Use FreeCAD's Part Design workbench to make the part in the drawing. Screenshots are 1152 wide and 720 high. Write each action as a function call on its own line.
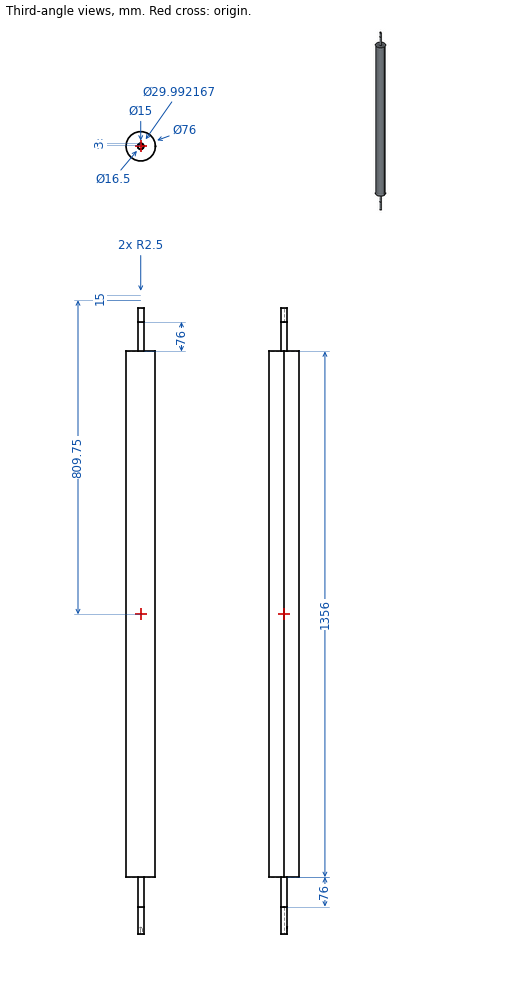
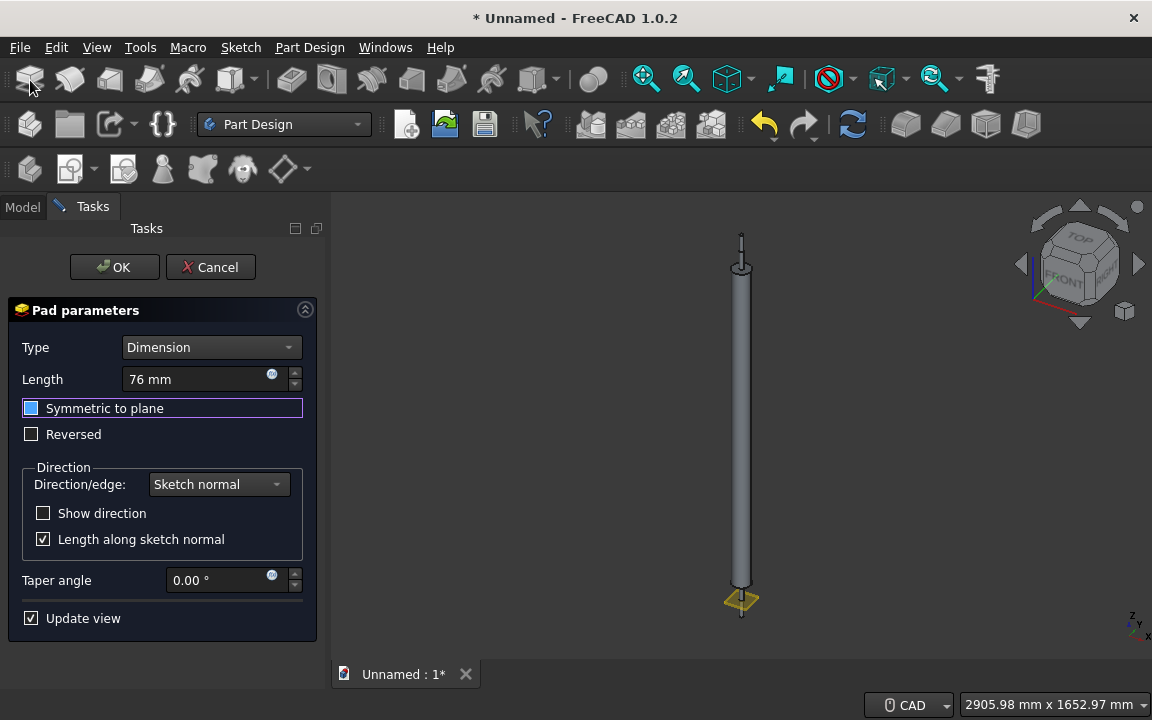
click(115, 267)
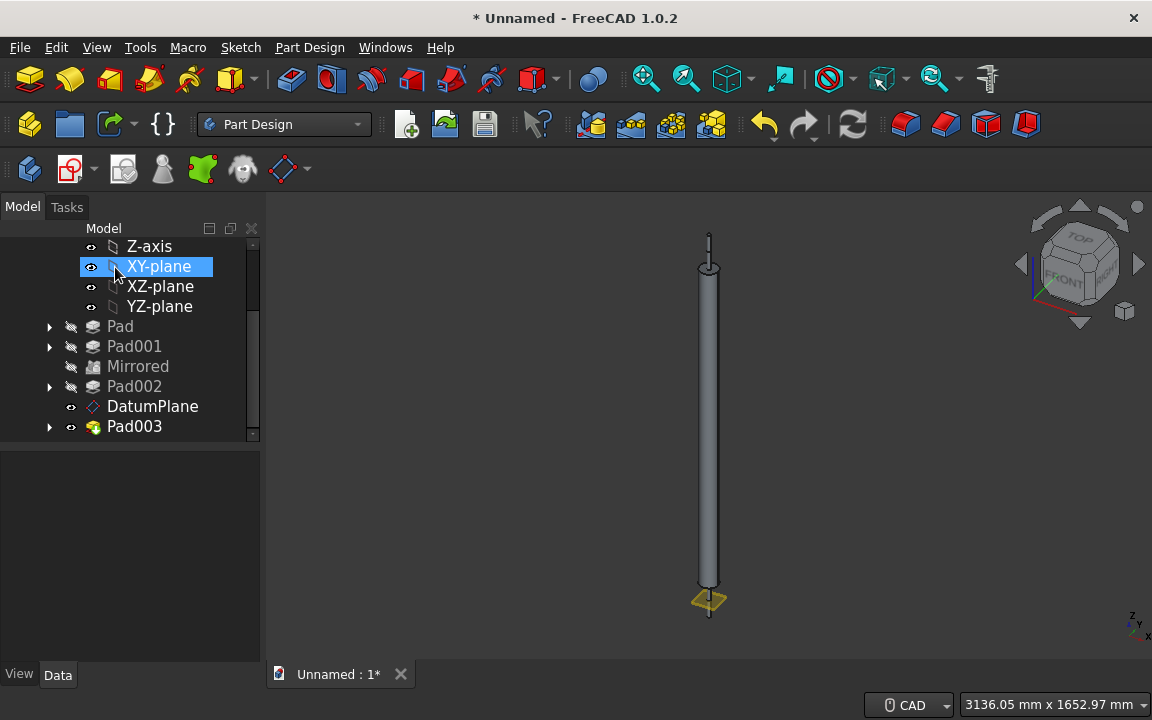
click(116, 407)
key(space)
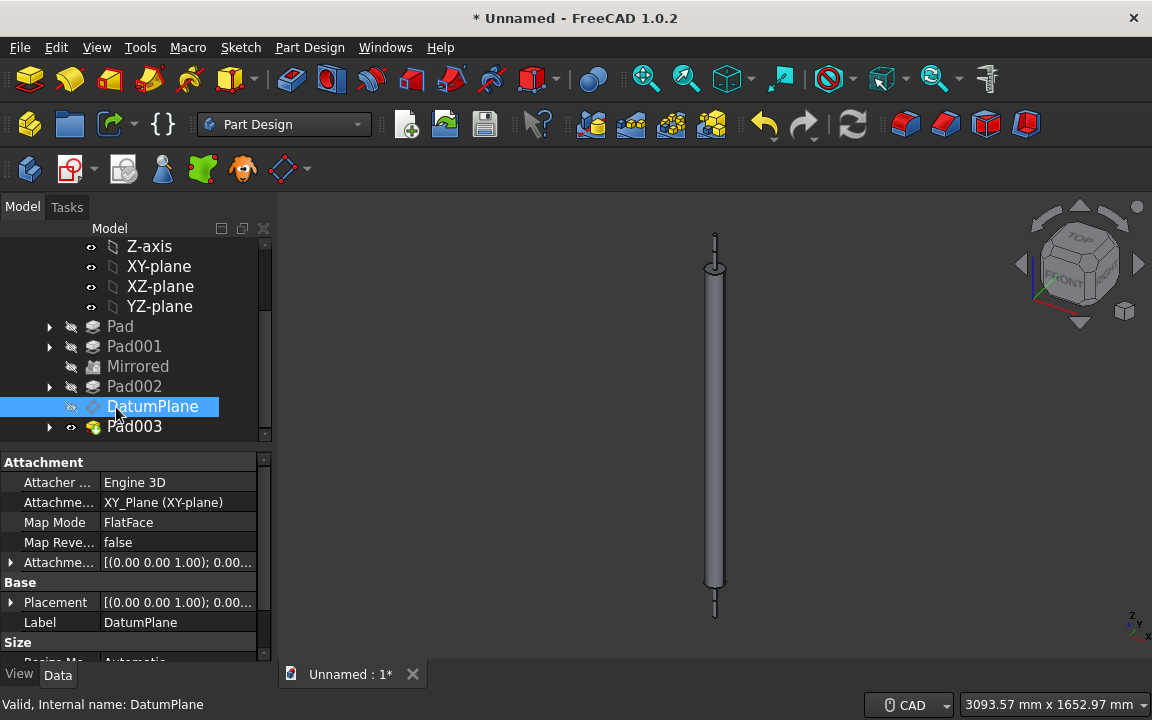
scroll(160, 342, down, 3)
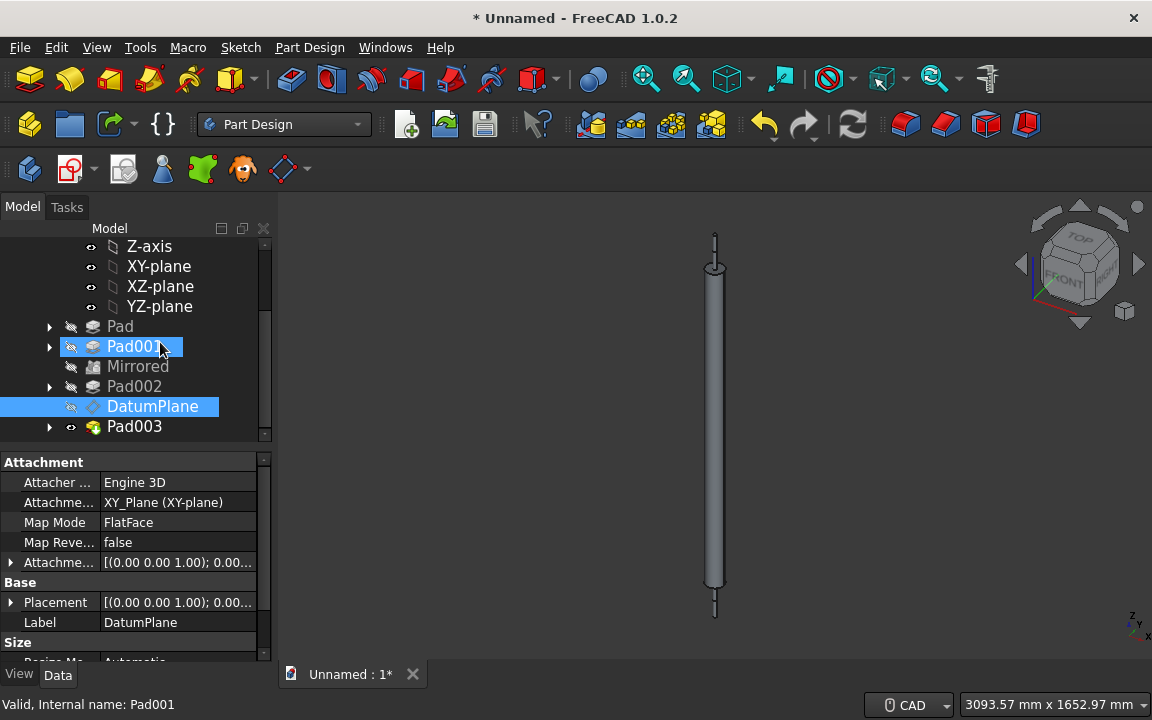
scroll(160, 342, up, 15)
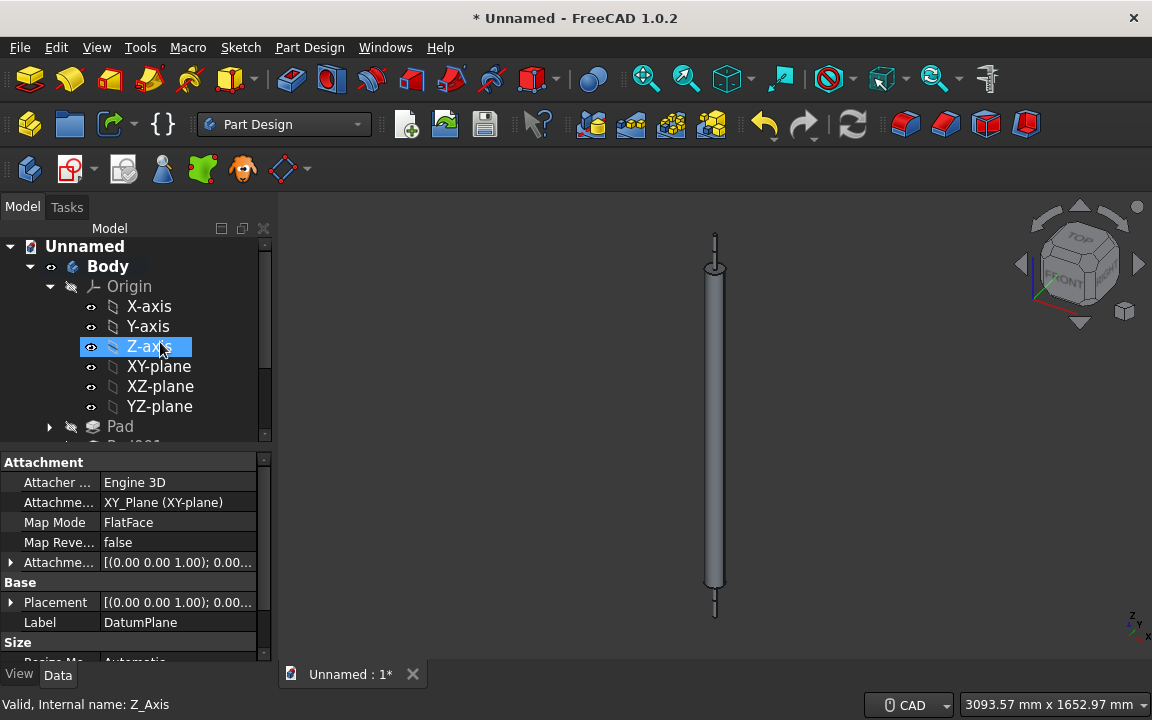
click(136, 387)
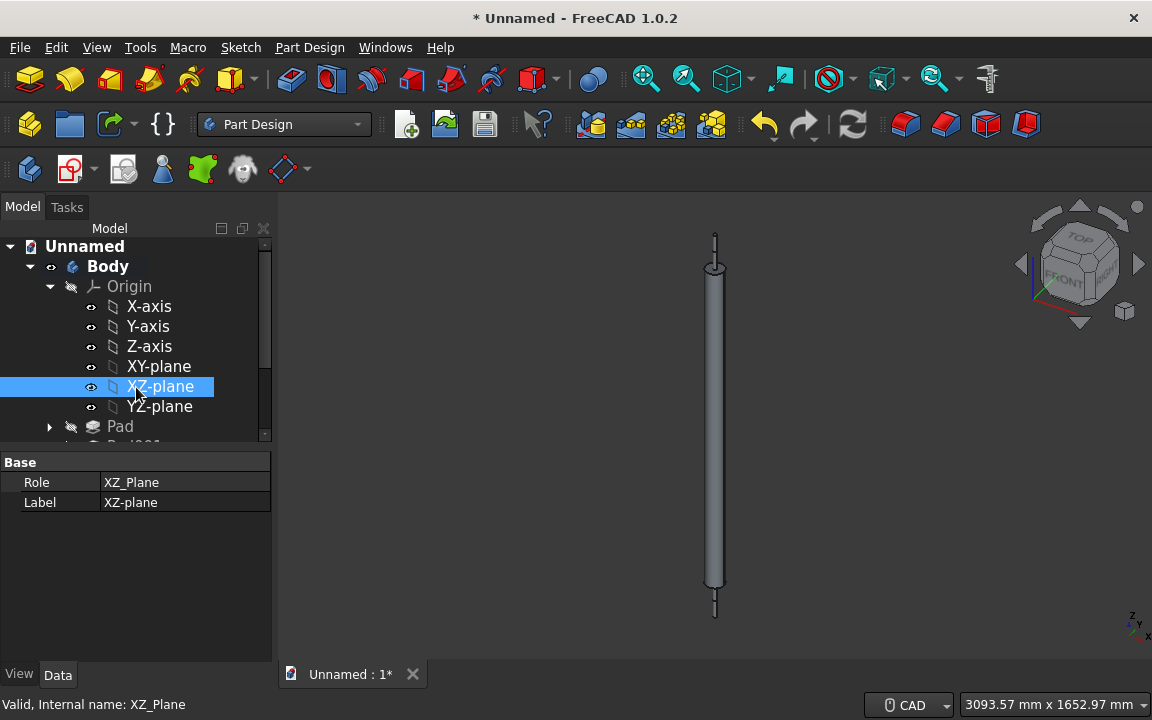
click(284, 170)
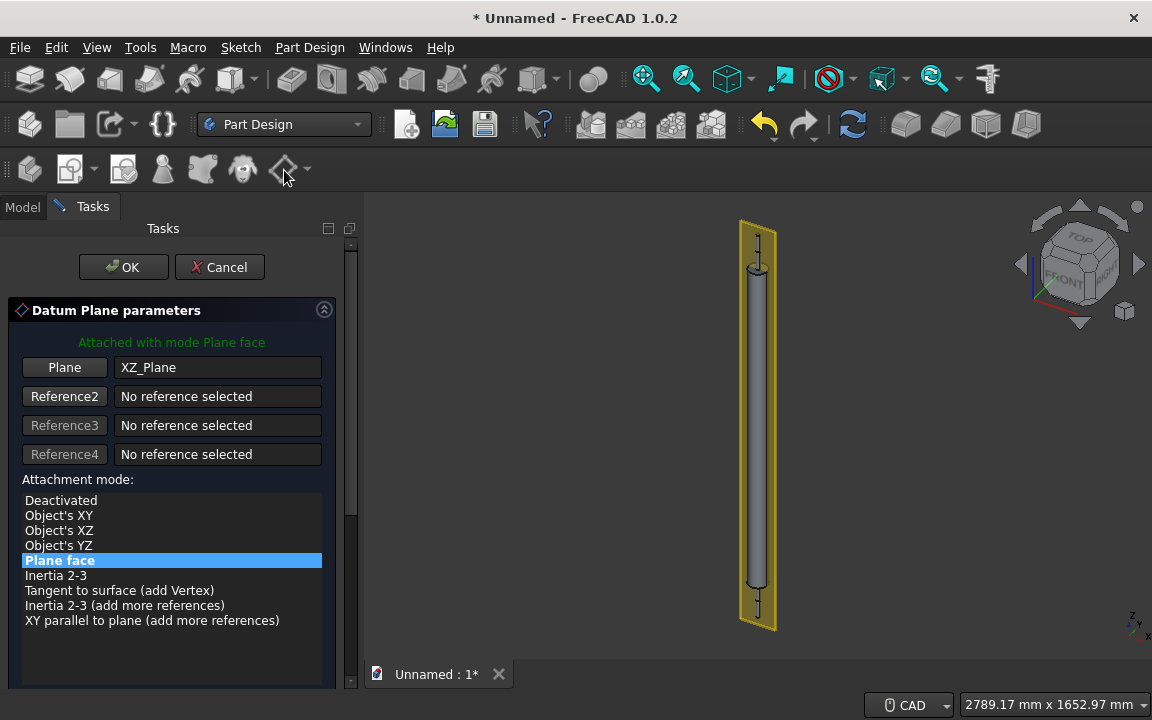
scroll(351, 463, down, 3)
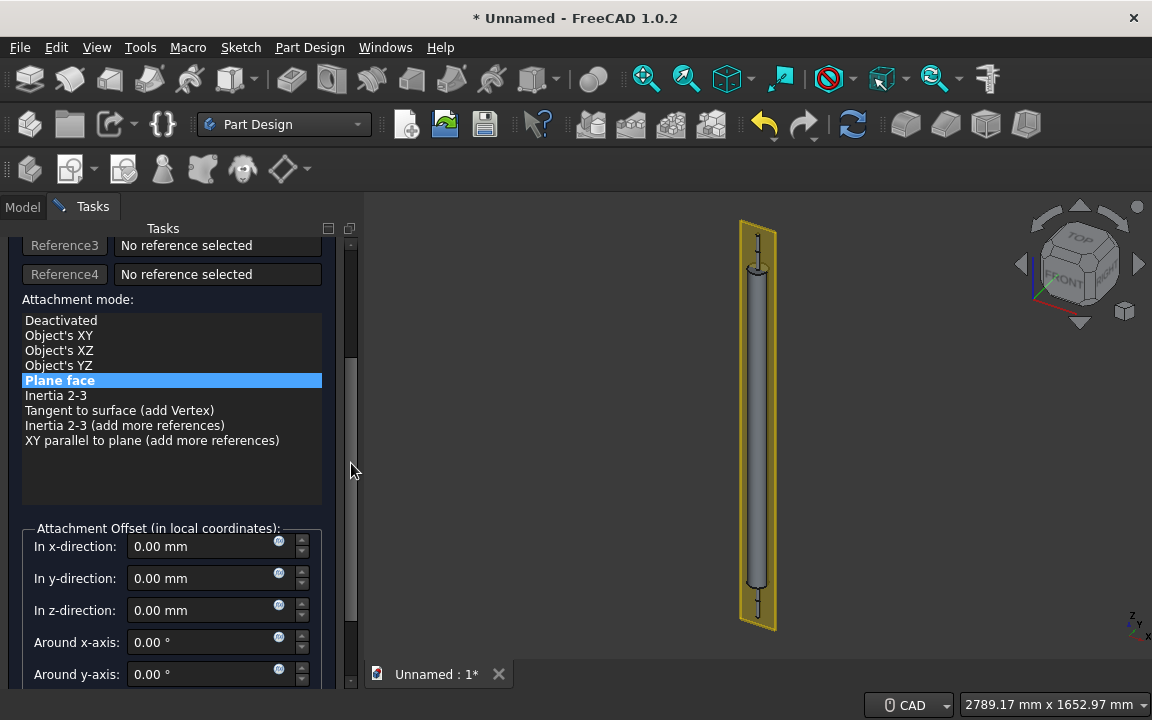
triple_click(210, 610)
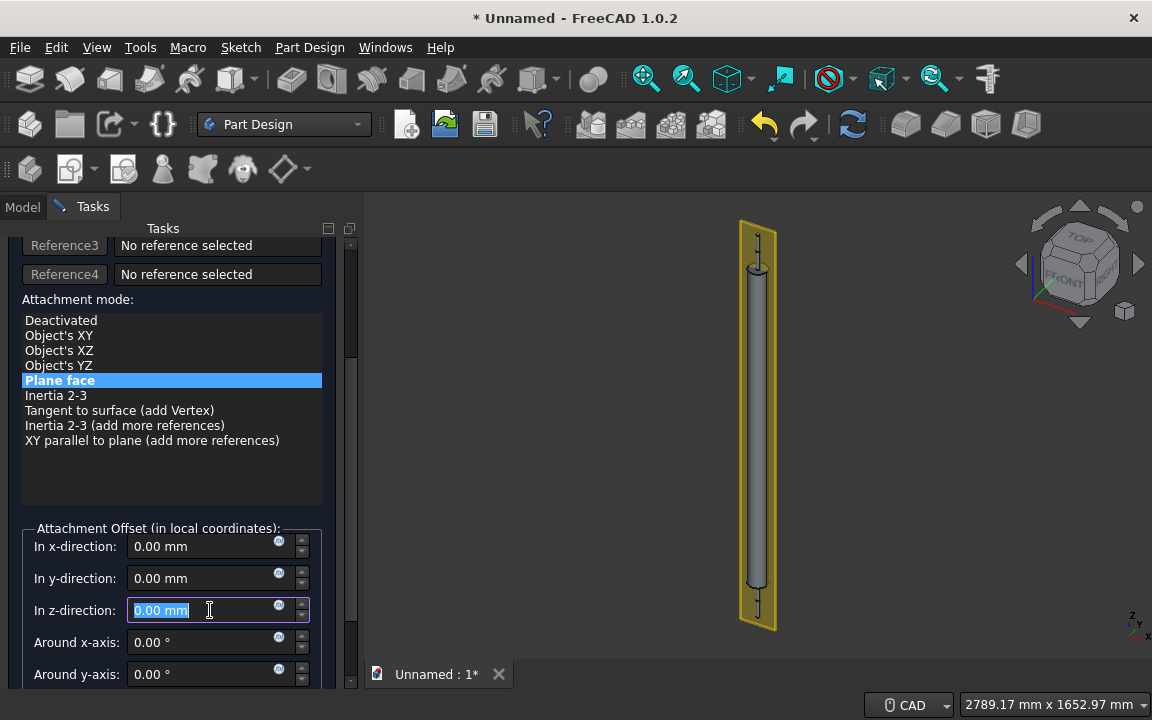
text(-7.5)
key(Tab)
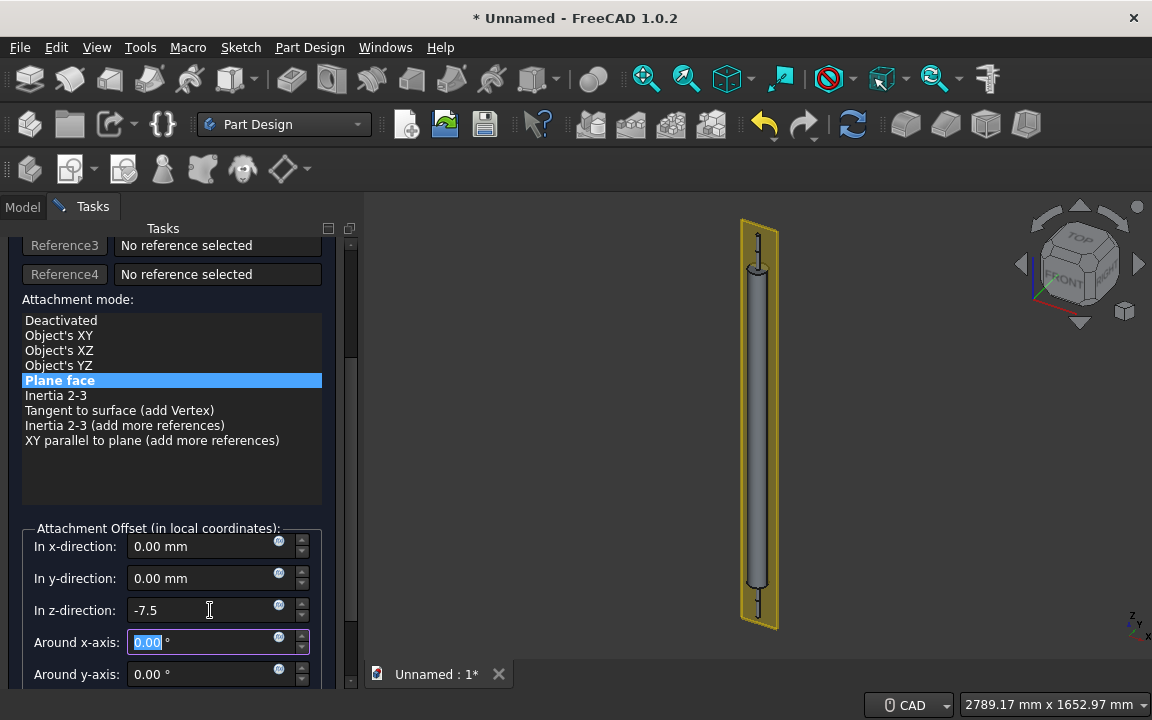
scroll(351, 463, up, 4)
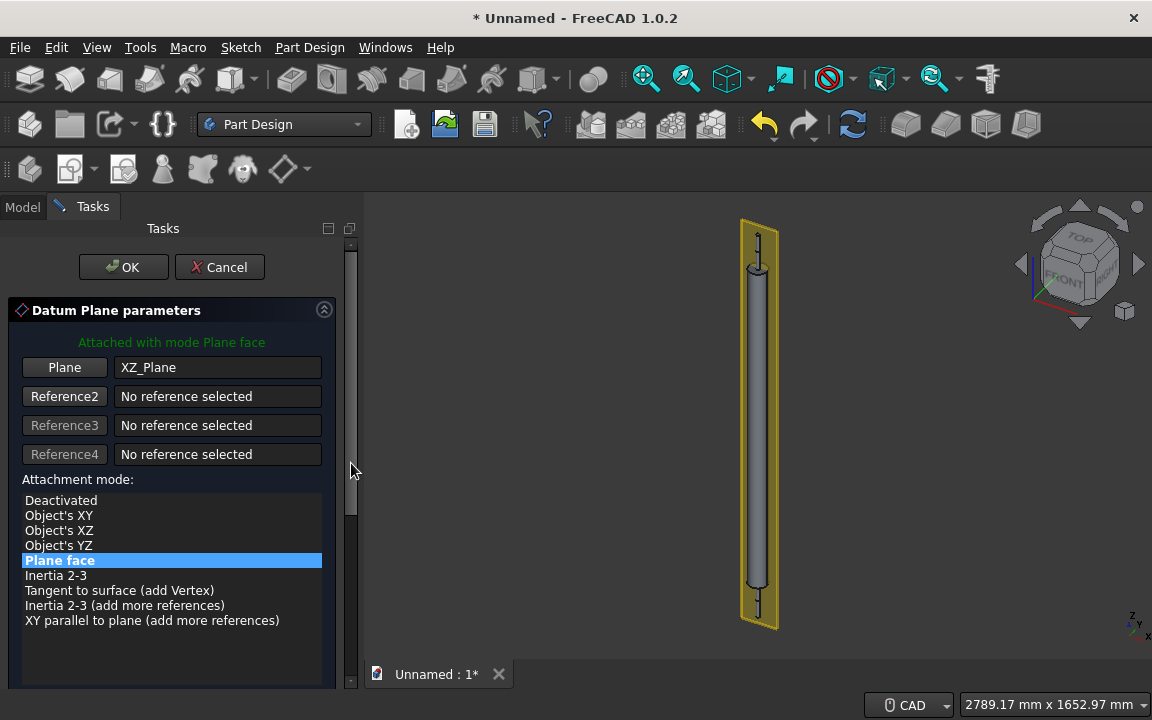
click(124, 267)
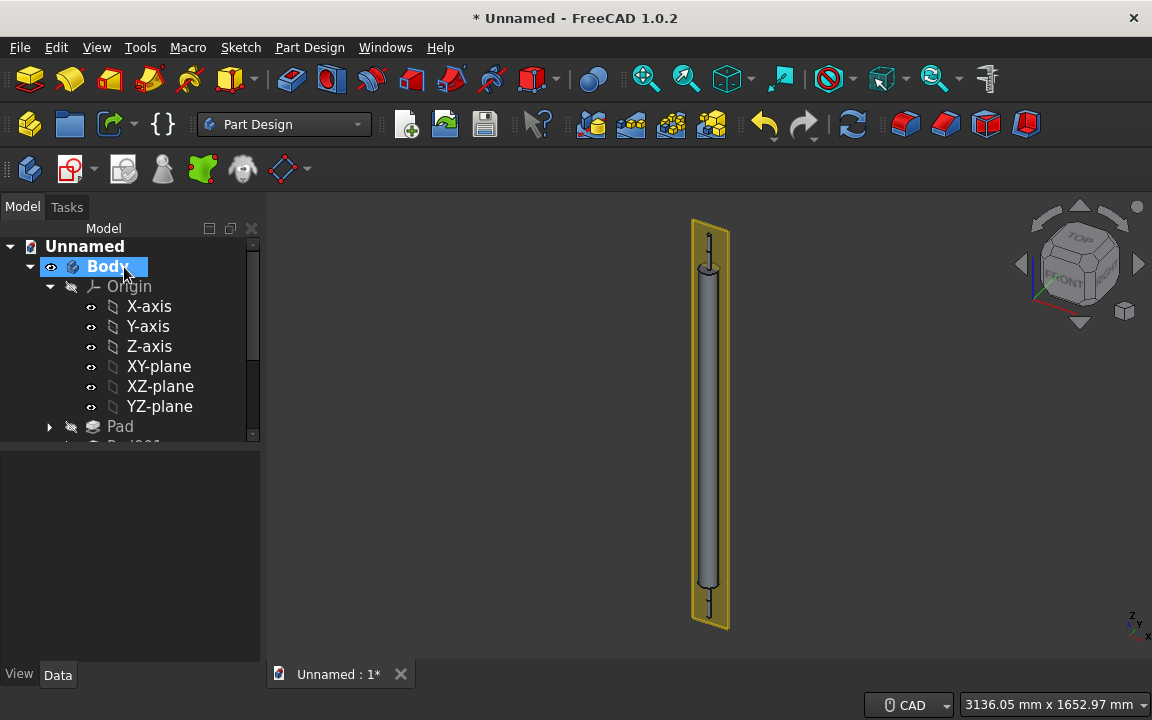
scroll(100, 342, down, 3)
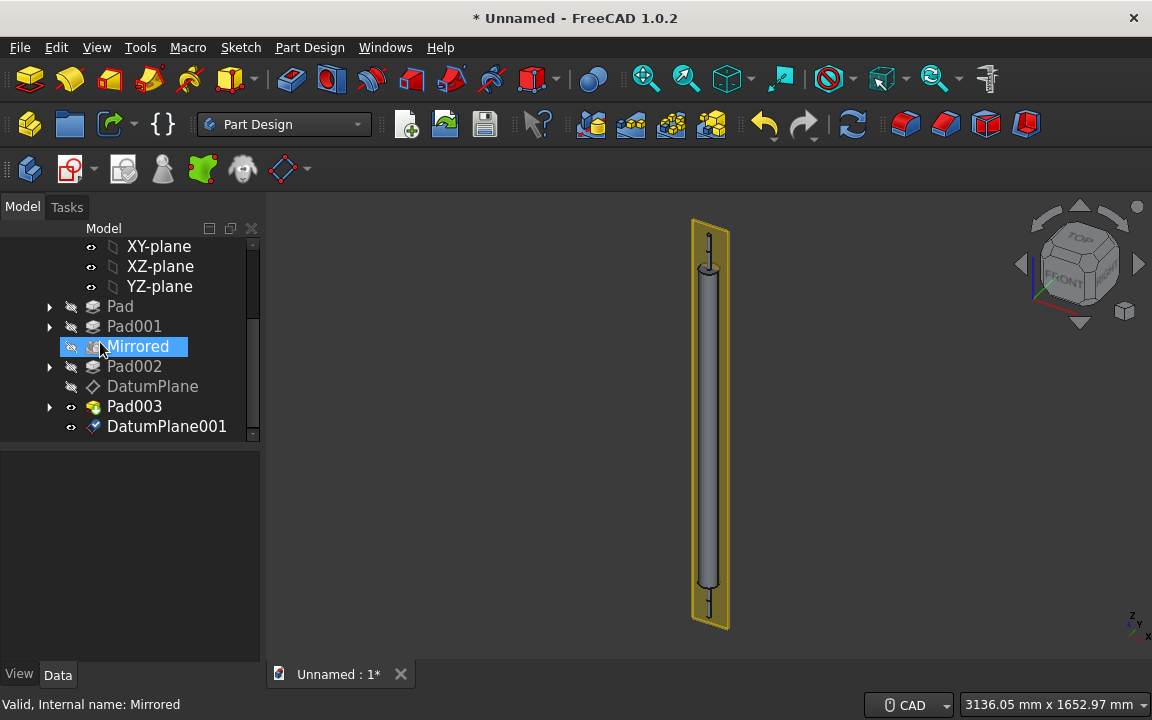
click(116, 427)